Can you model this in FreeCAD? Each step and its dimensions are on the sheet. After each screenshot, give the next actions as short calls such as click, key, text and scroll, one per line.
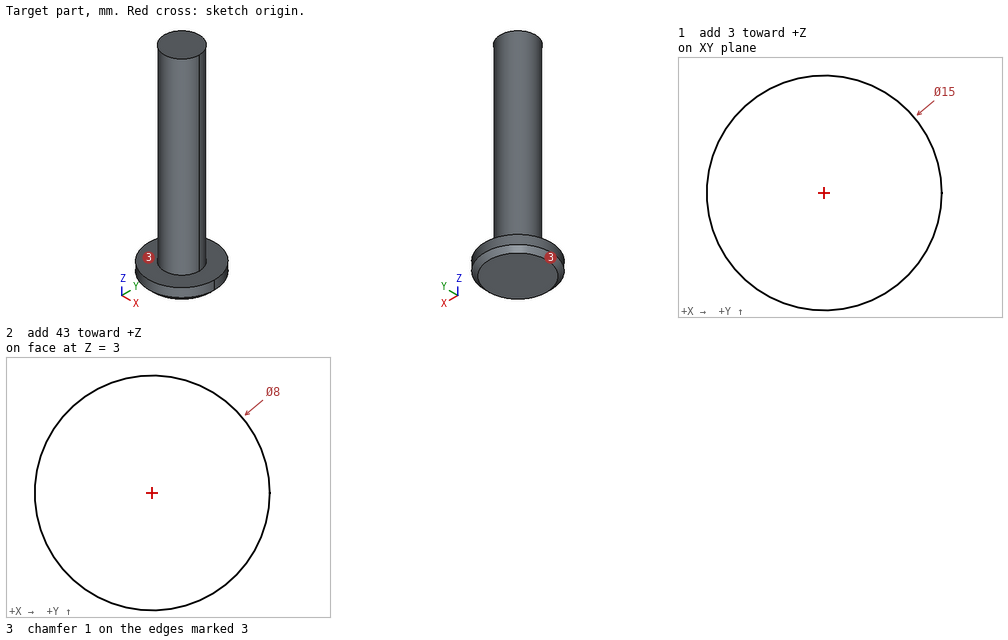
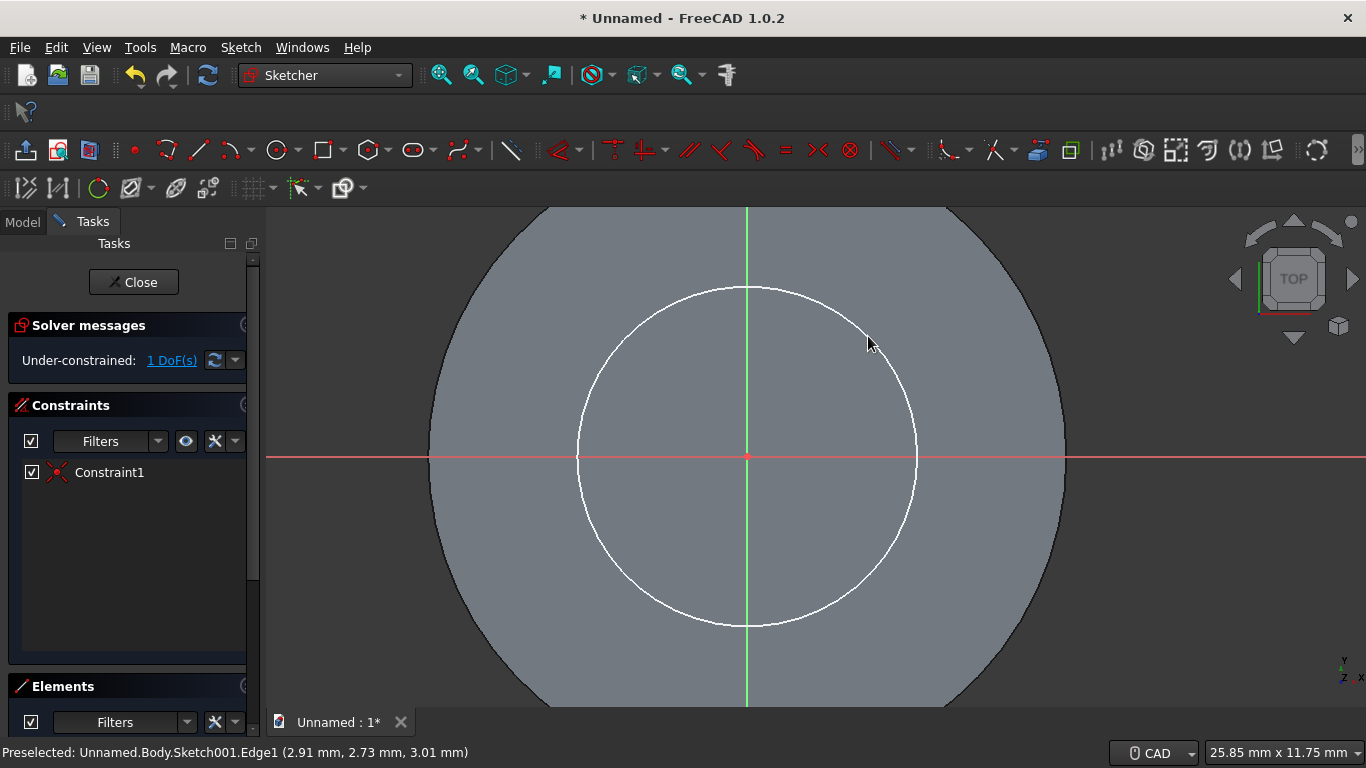
key(d)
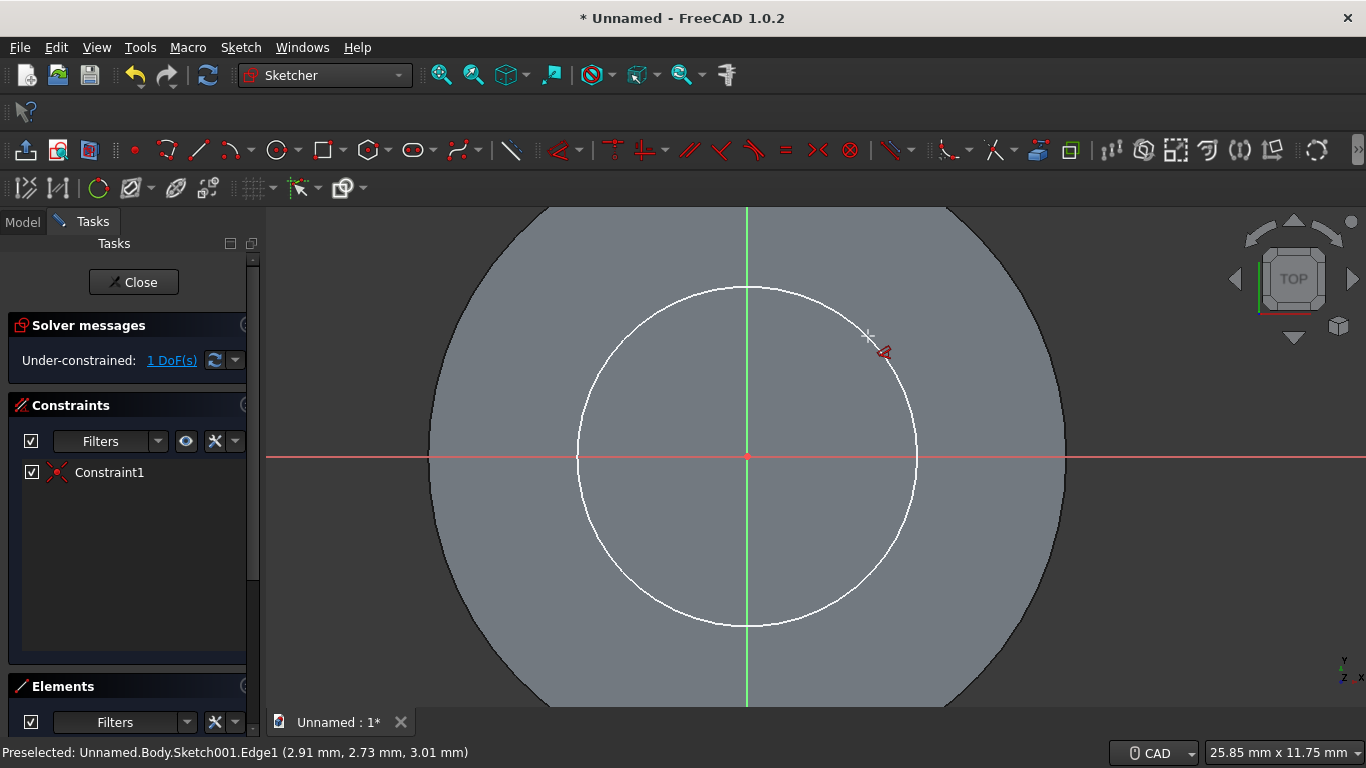
click(867, 336)
click(890, 313)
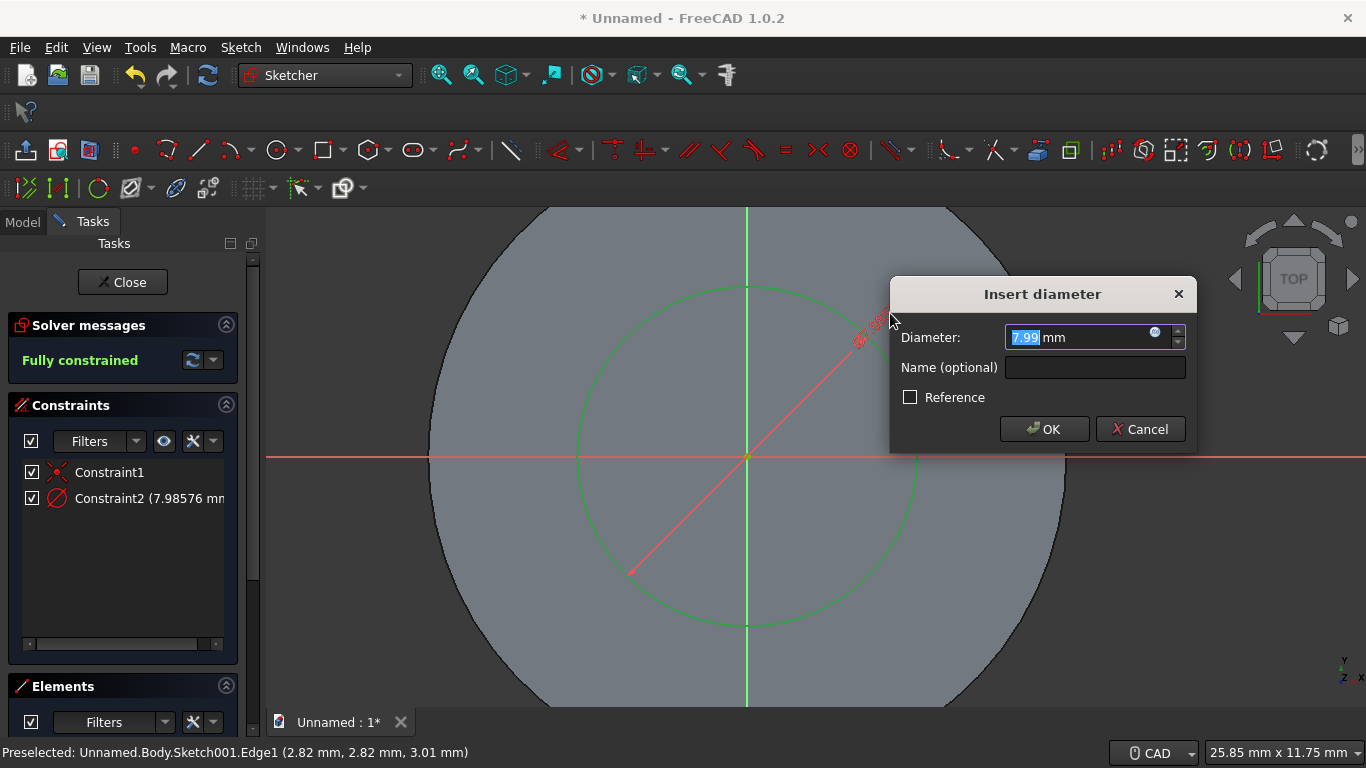
text(8)
key(Return)
key(Escape)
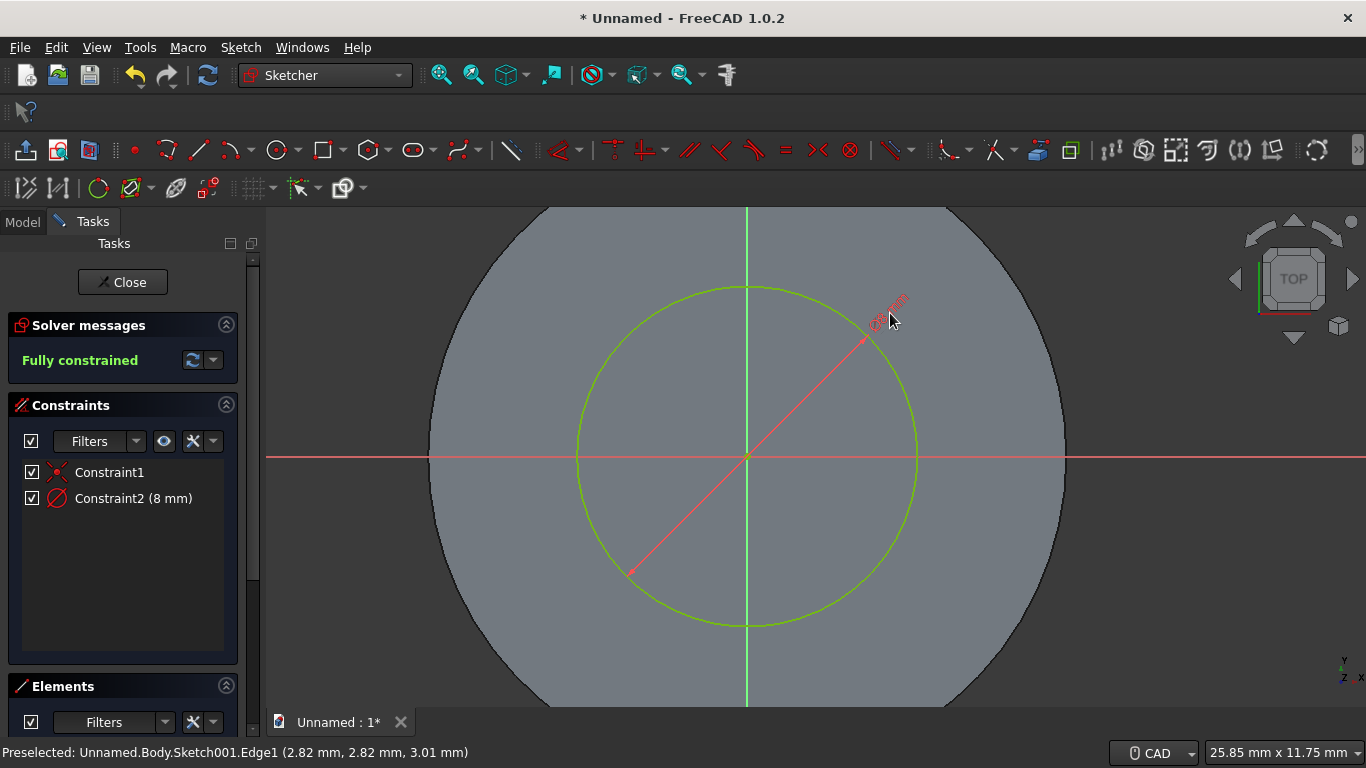
click(123, 282)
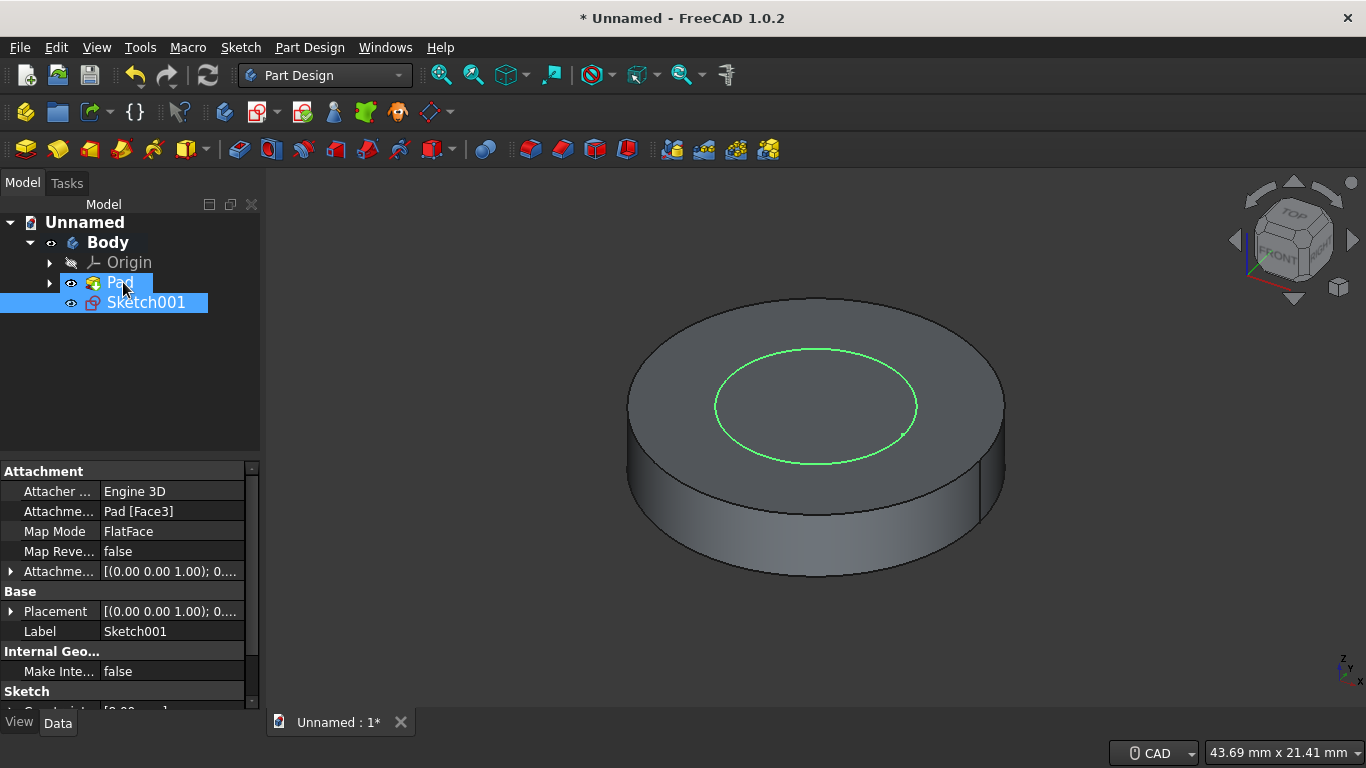
click(26, 150)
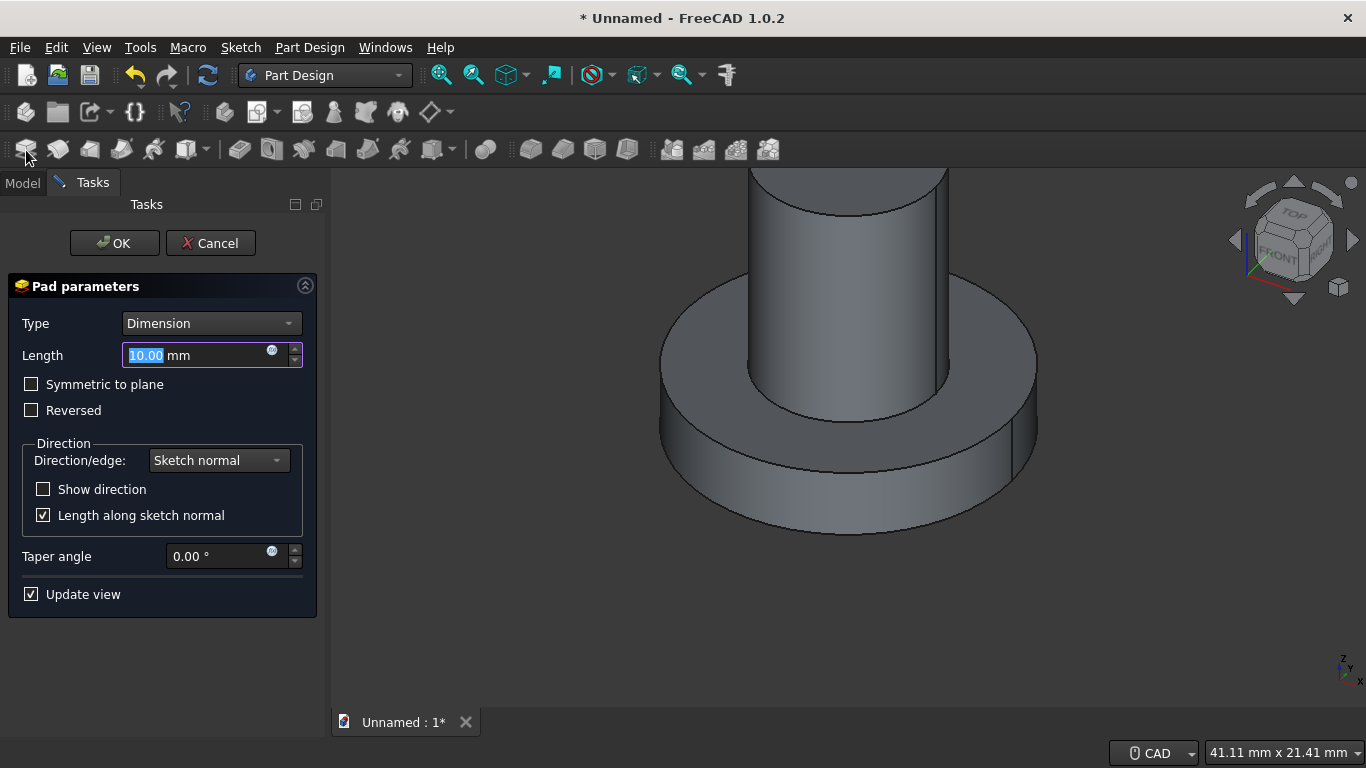
text(43)
key(Tab)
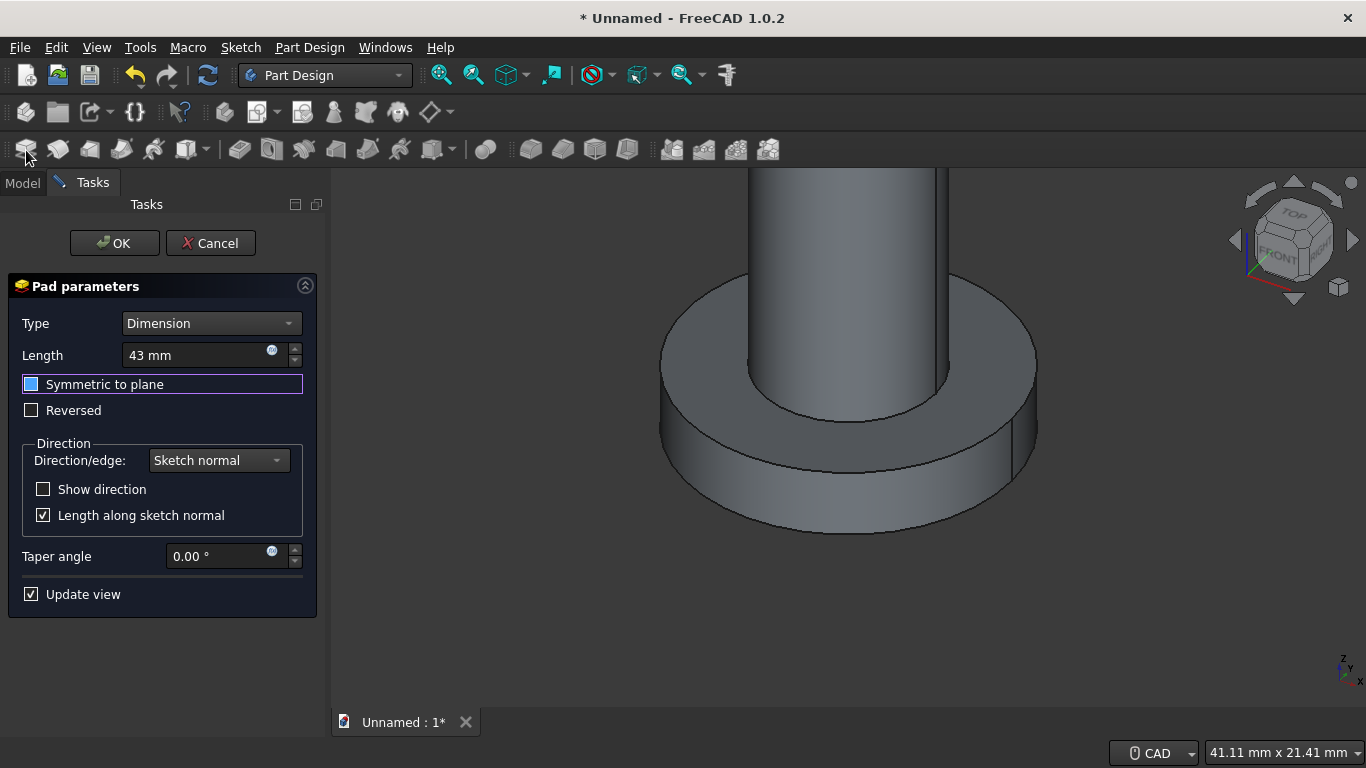
click(115, 243)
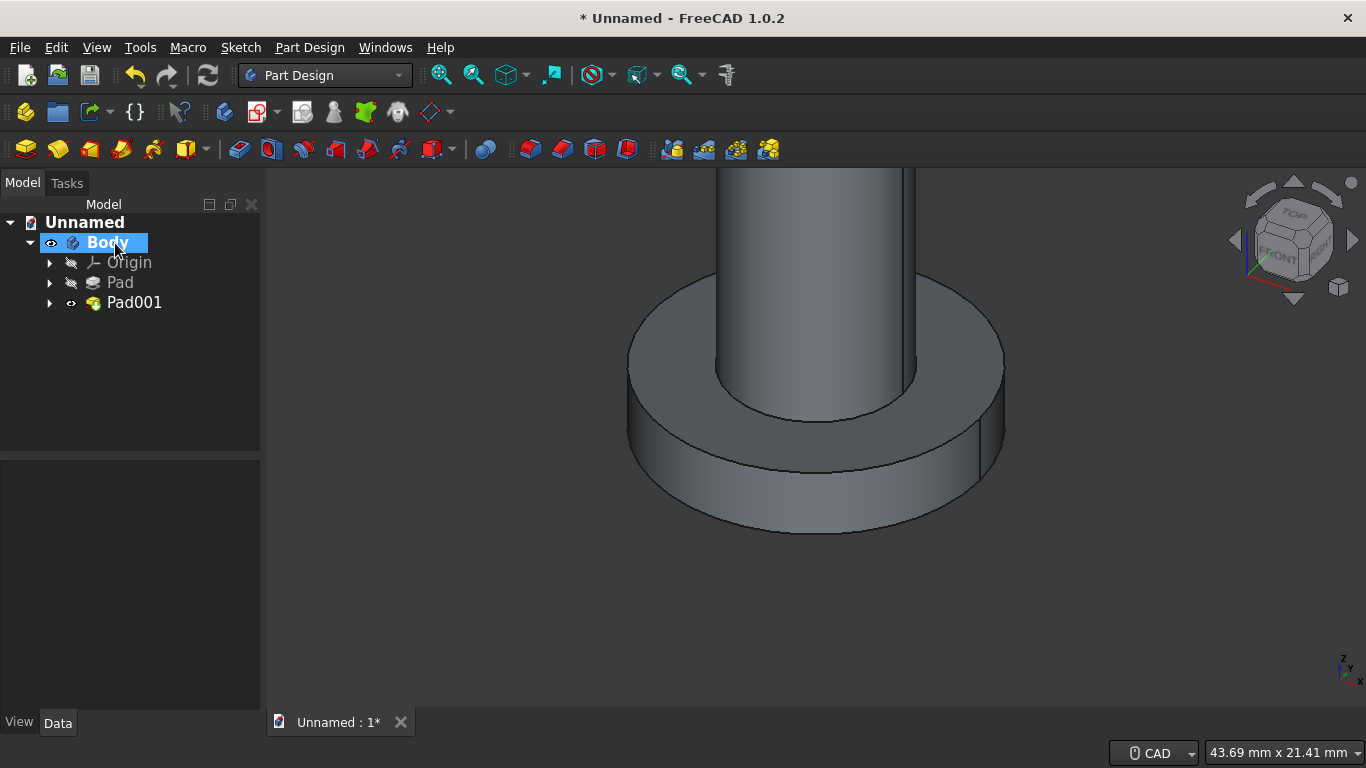
click(442, 76)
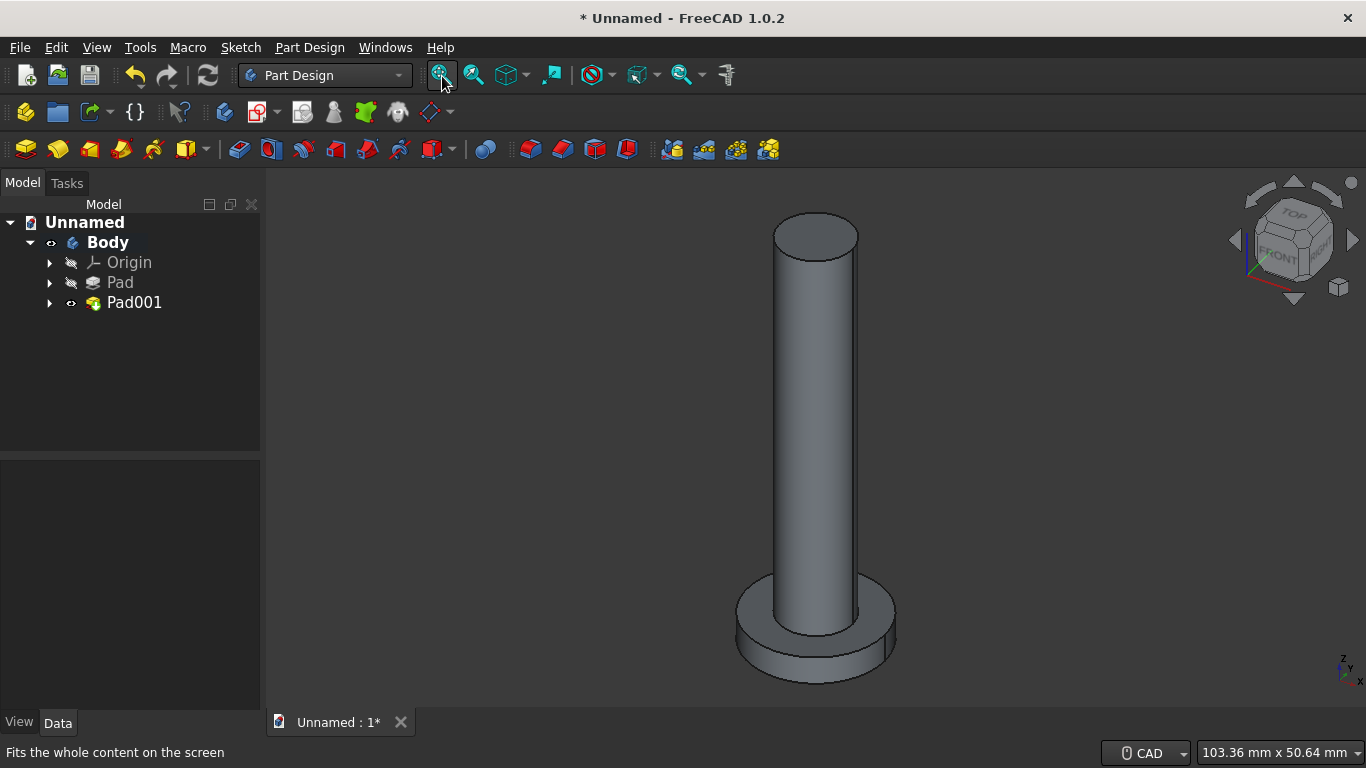
key(0)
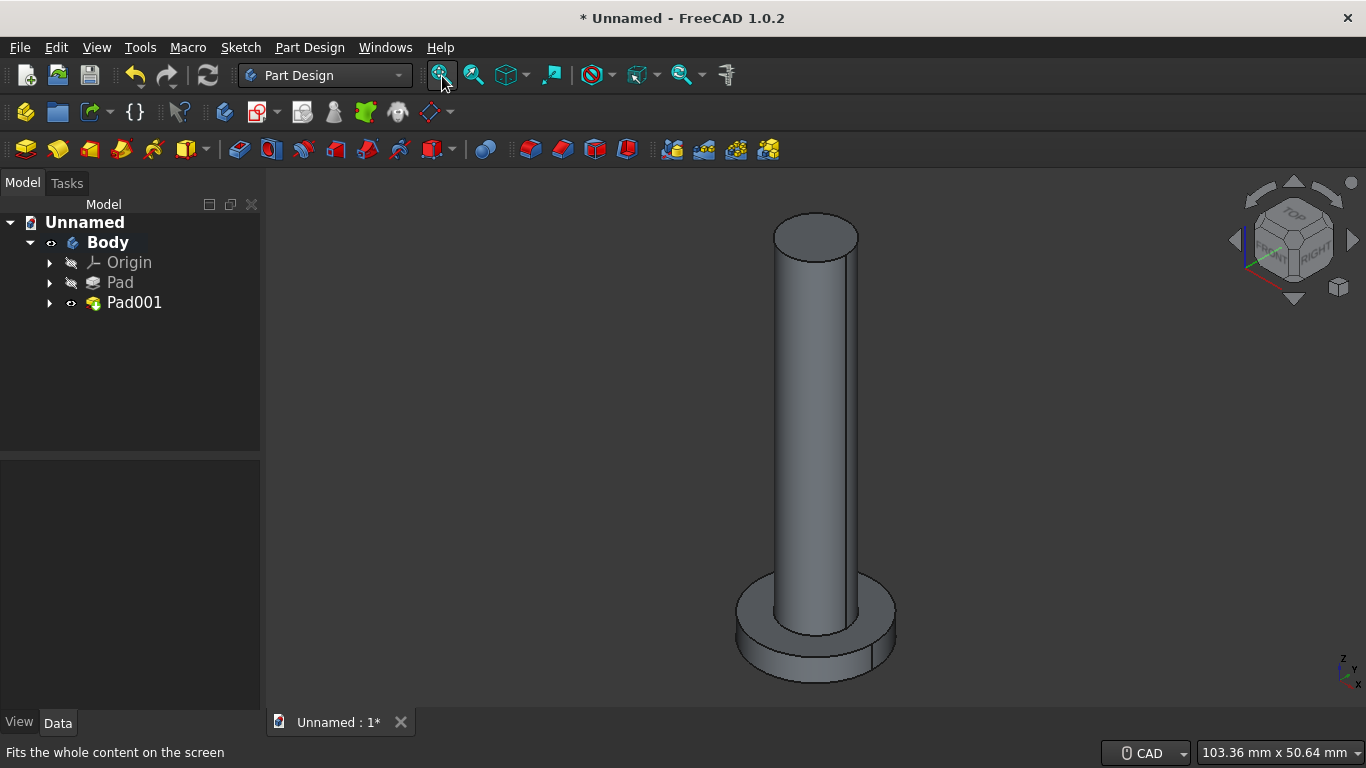
key(2)